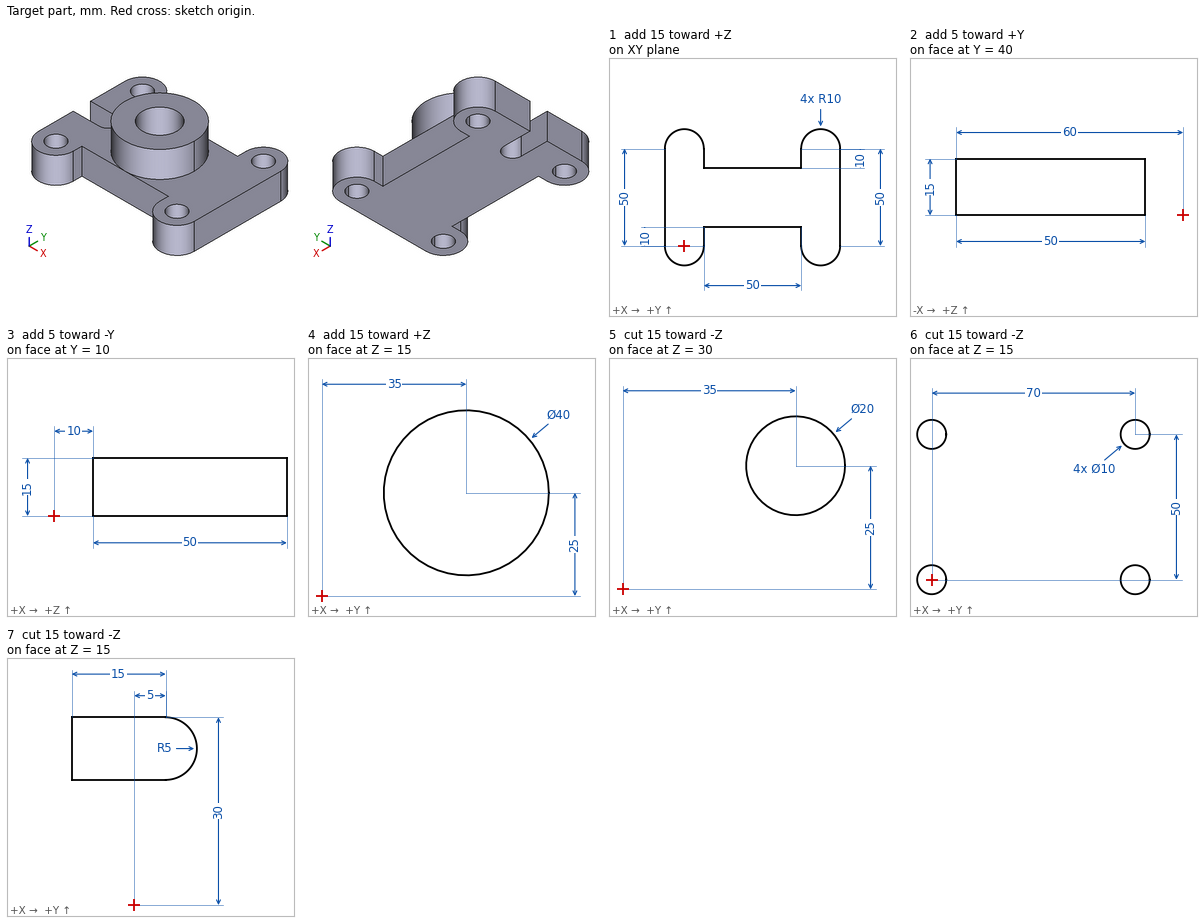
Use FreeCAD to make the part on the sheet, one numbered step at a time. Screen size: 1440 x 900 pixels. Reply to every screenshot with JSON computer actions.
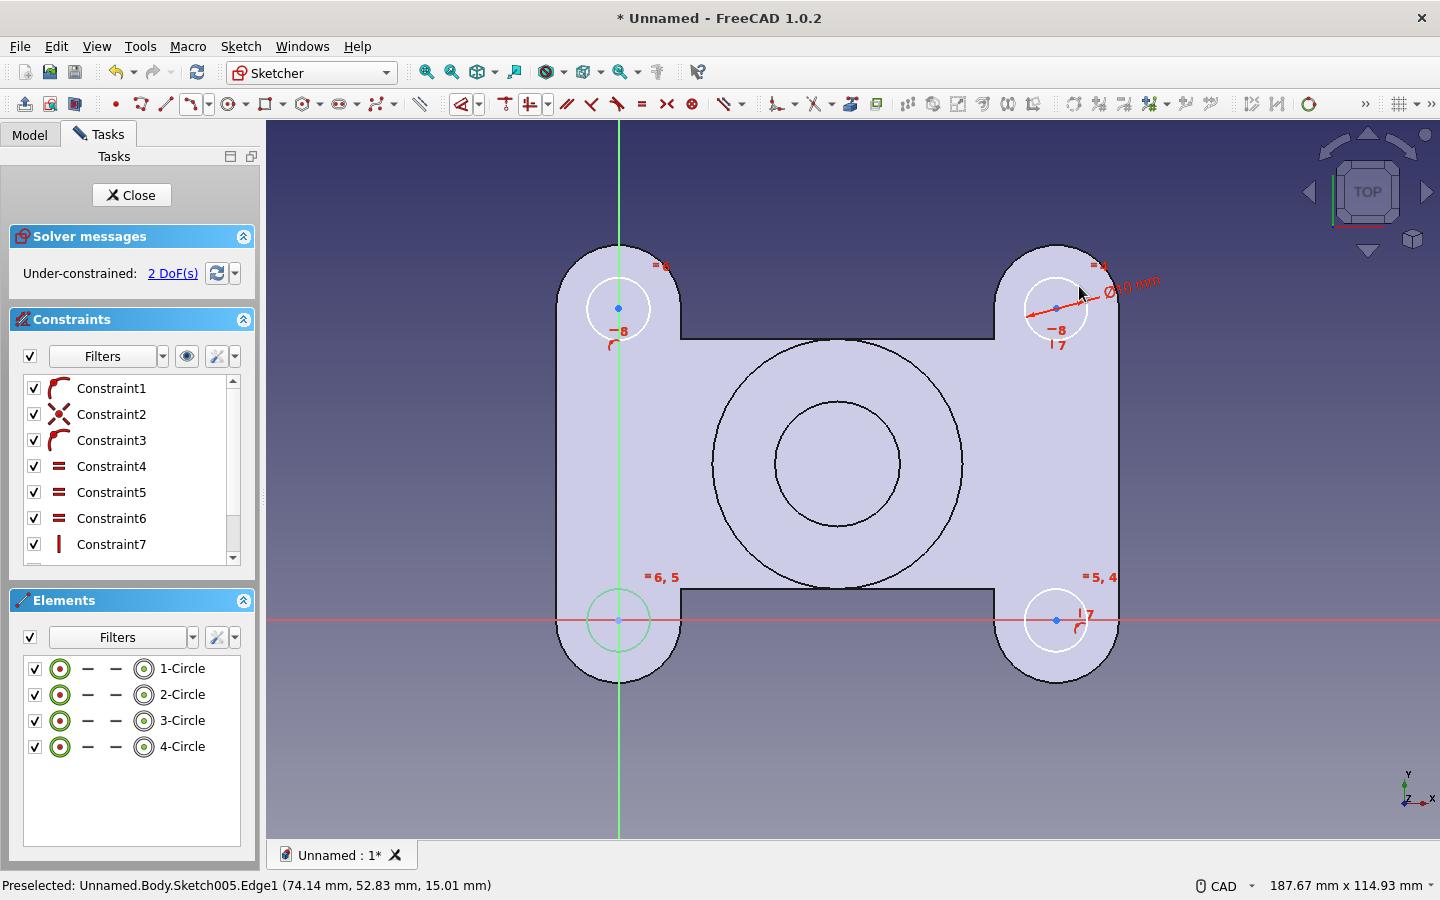
{"action": "left_click", "coordinate": [1056, 309]}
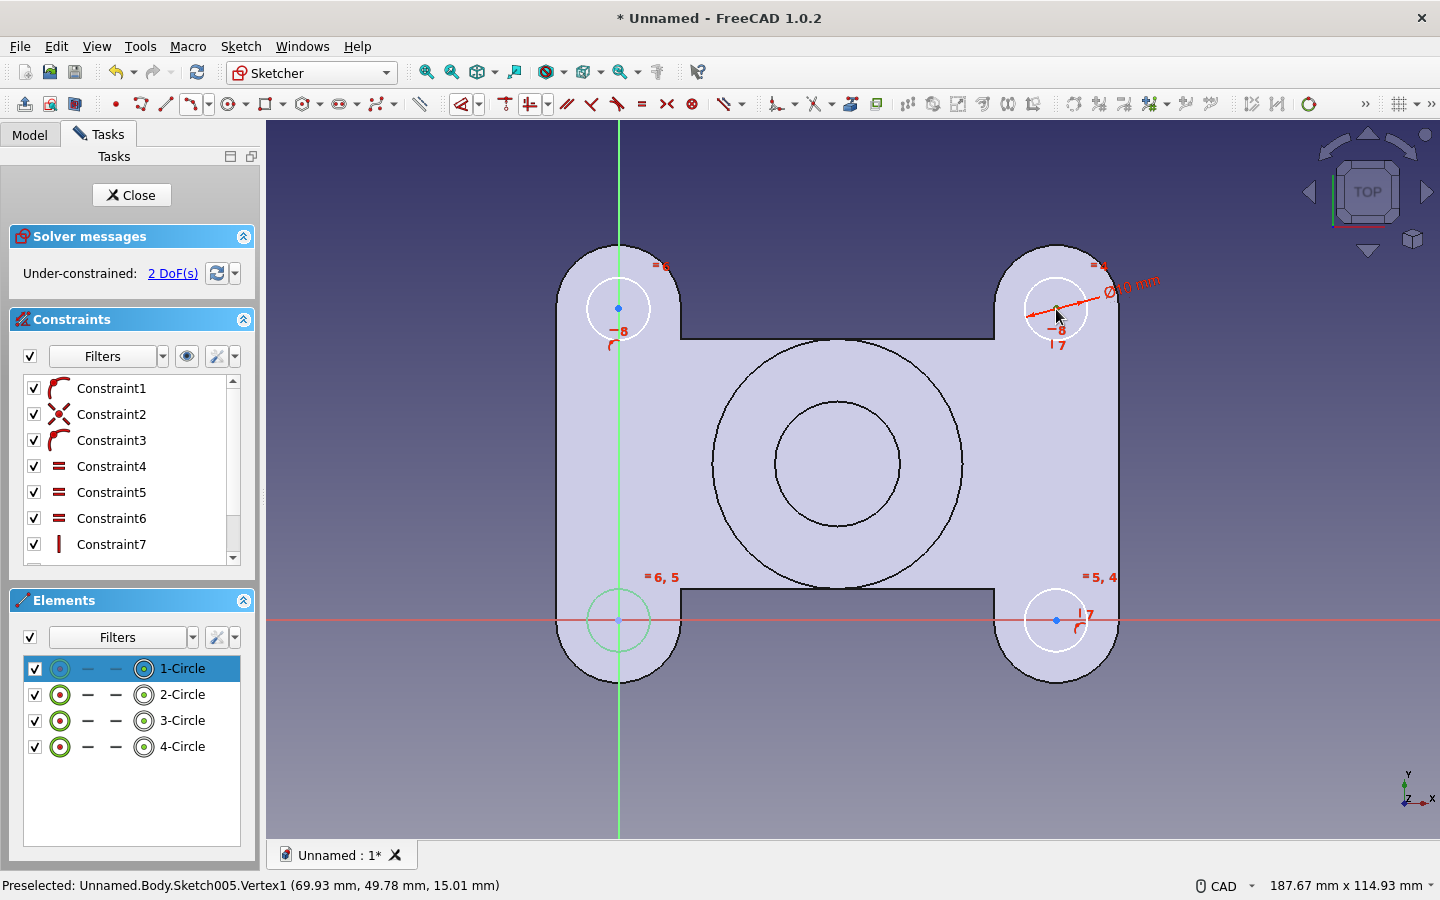
{"action": "left_click", "coordinate": [478, 104]}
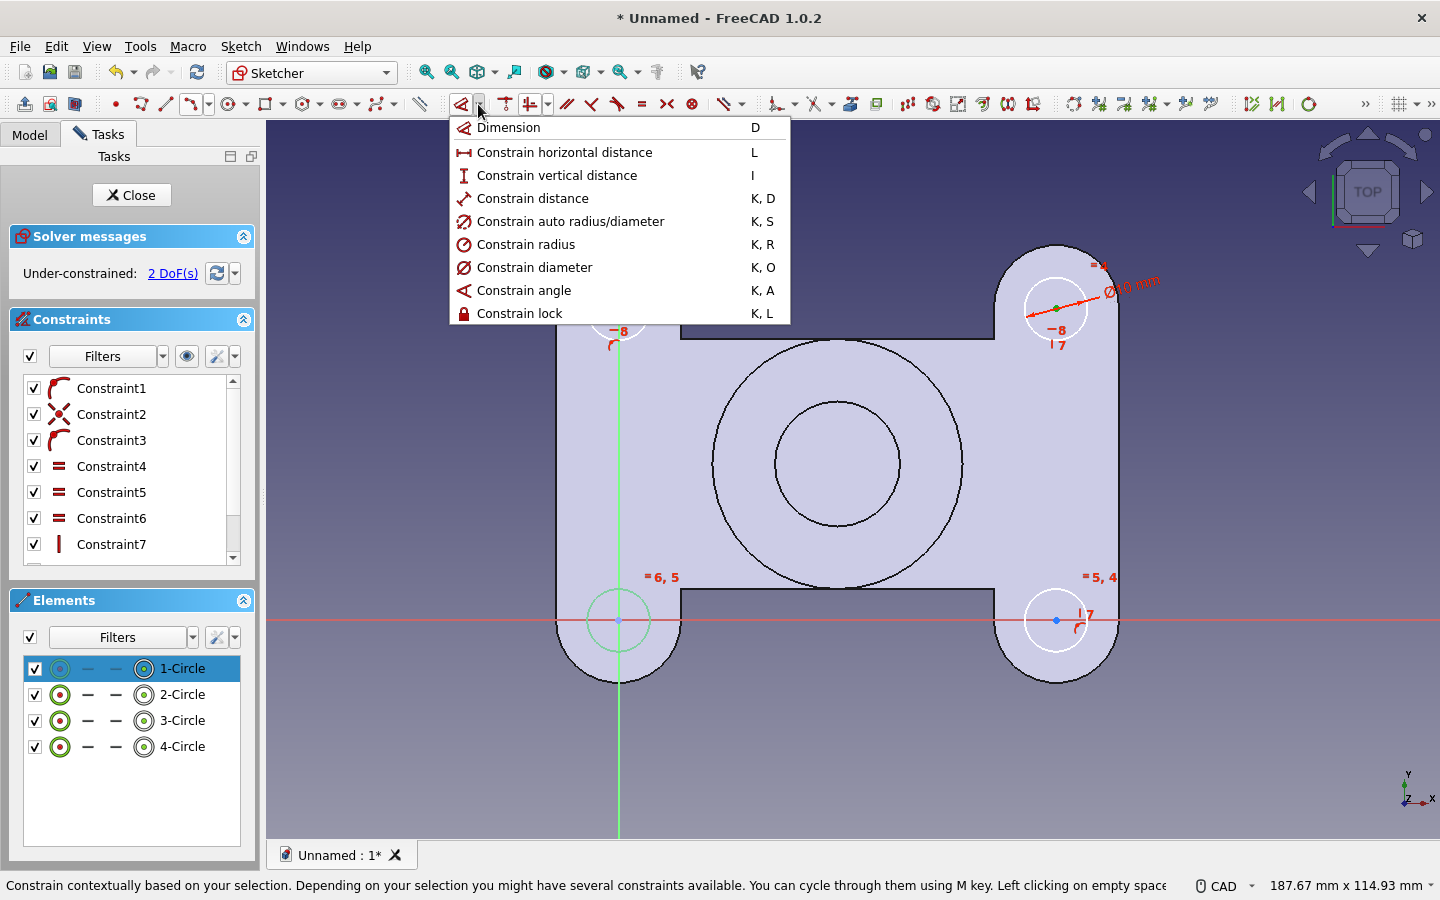
{"action": "left_click", "coordinate": [620, 152]}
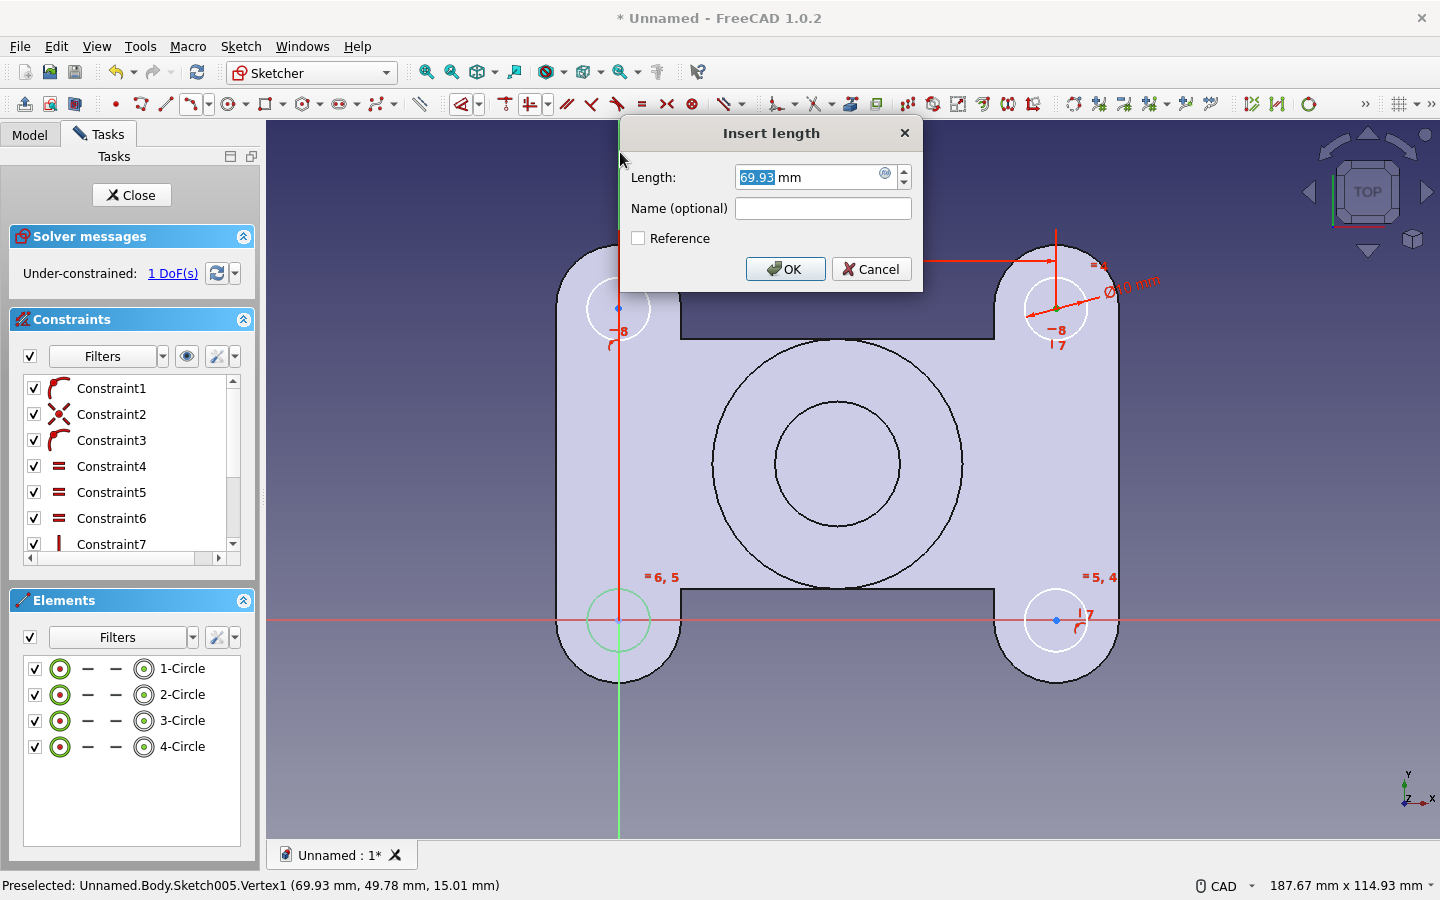
{"action": "type", "text": "70"}
{"action": "key", "text": "Return"}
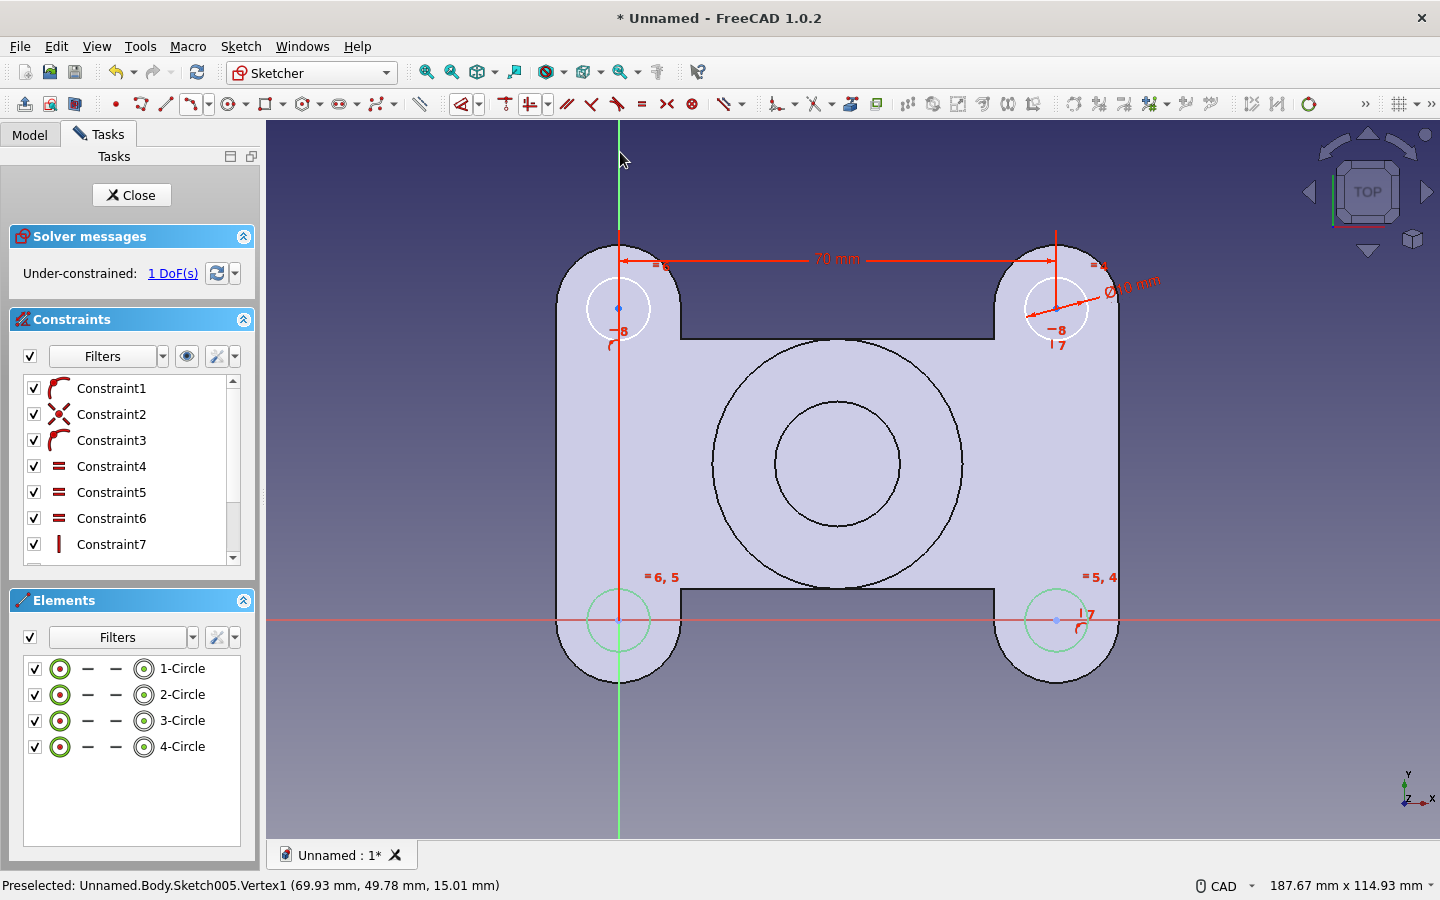
{"action": "left_click", "coordinate": [1056, 309]}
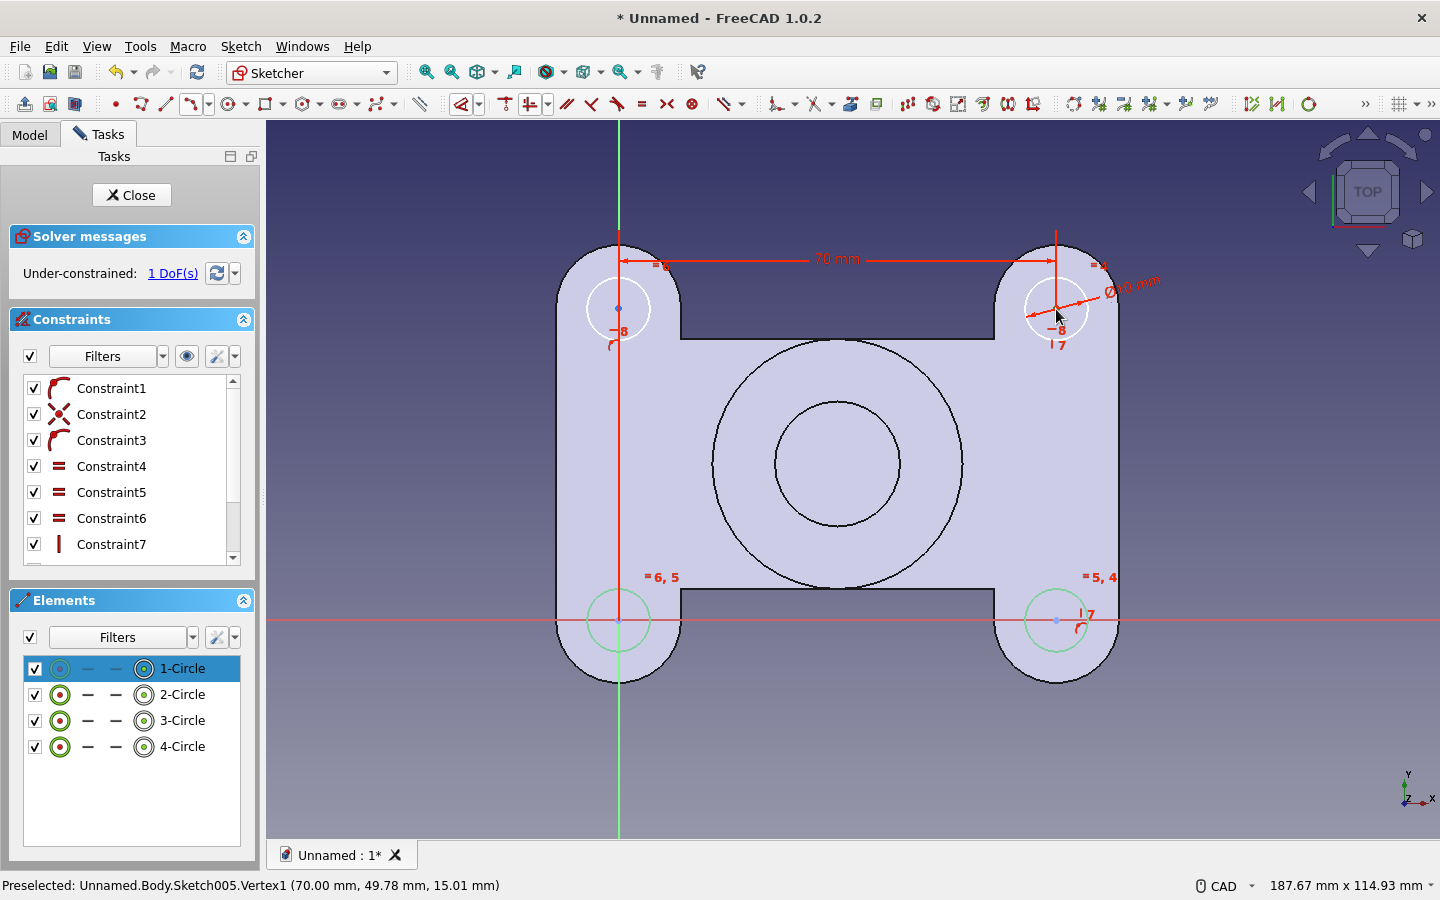
{"action": "key", "text": "i"}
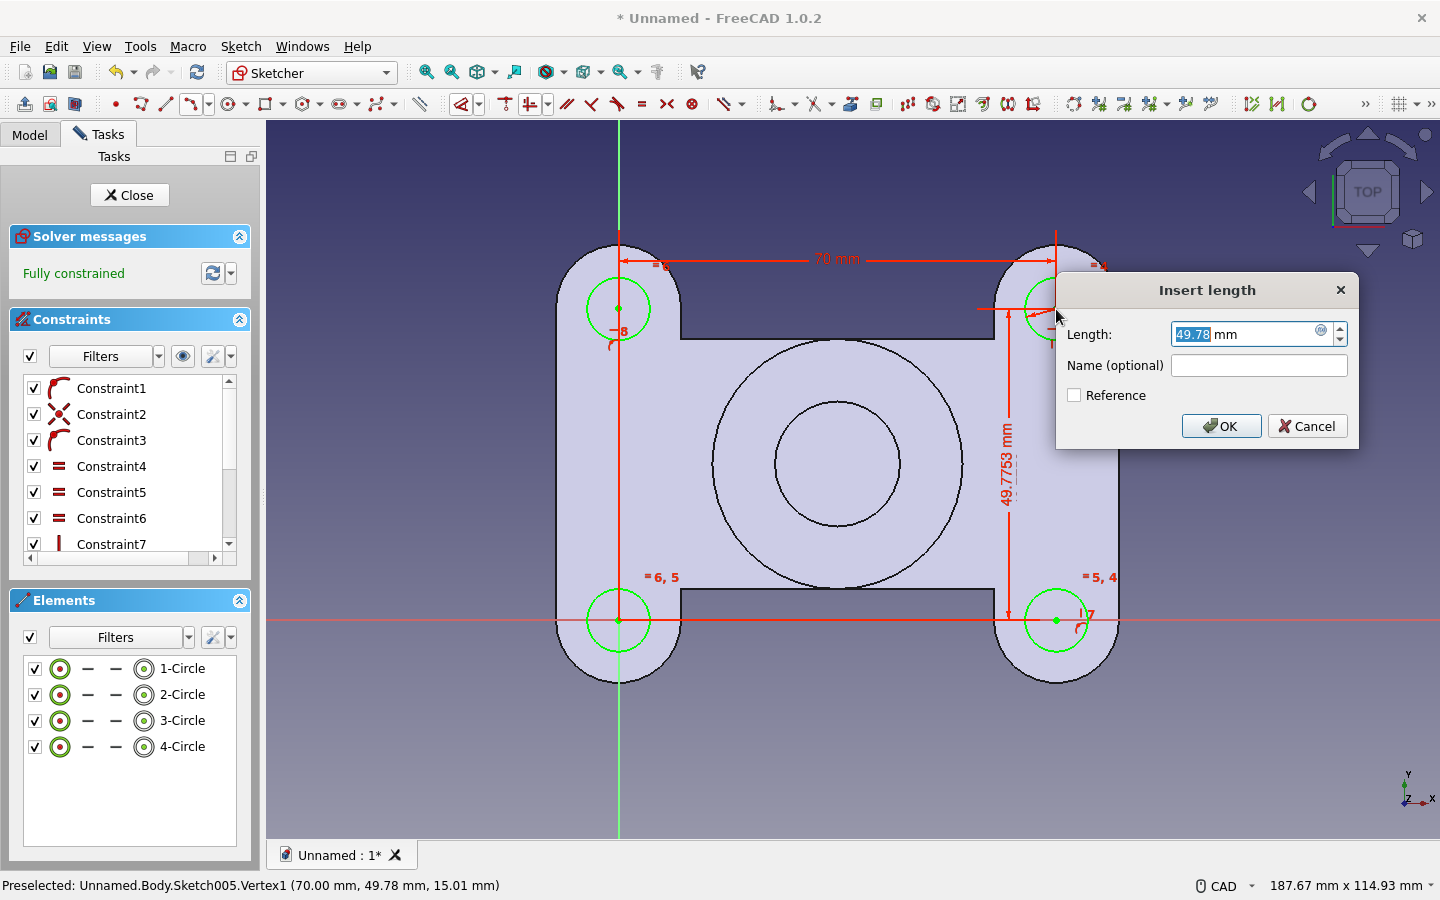
{"action": "type", "text": "50"}
{"action": "key", "text": "Return"}